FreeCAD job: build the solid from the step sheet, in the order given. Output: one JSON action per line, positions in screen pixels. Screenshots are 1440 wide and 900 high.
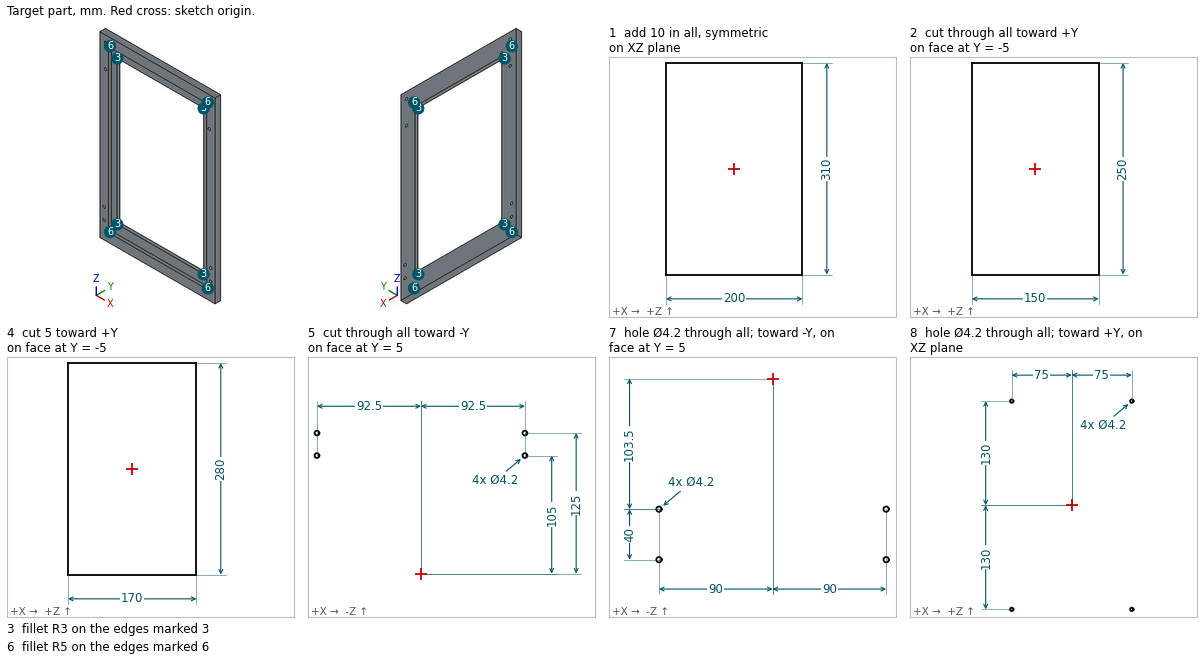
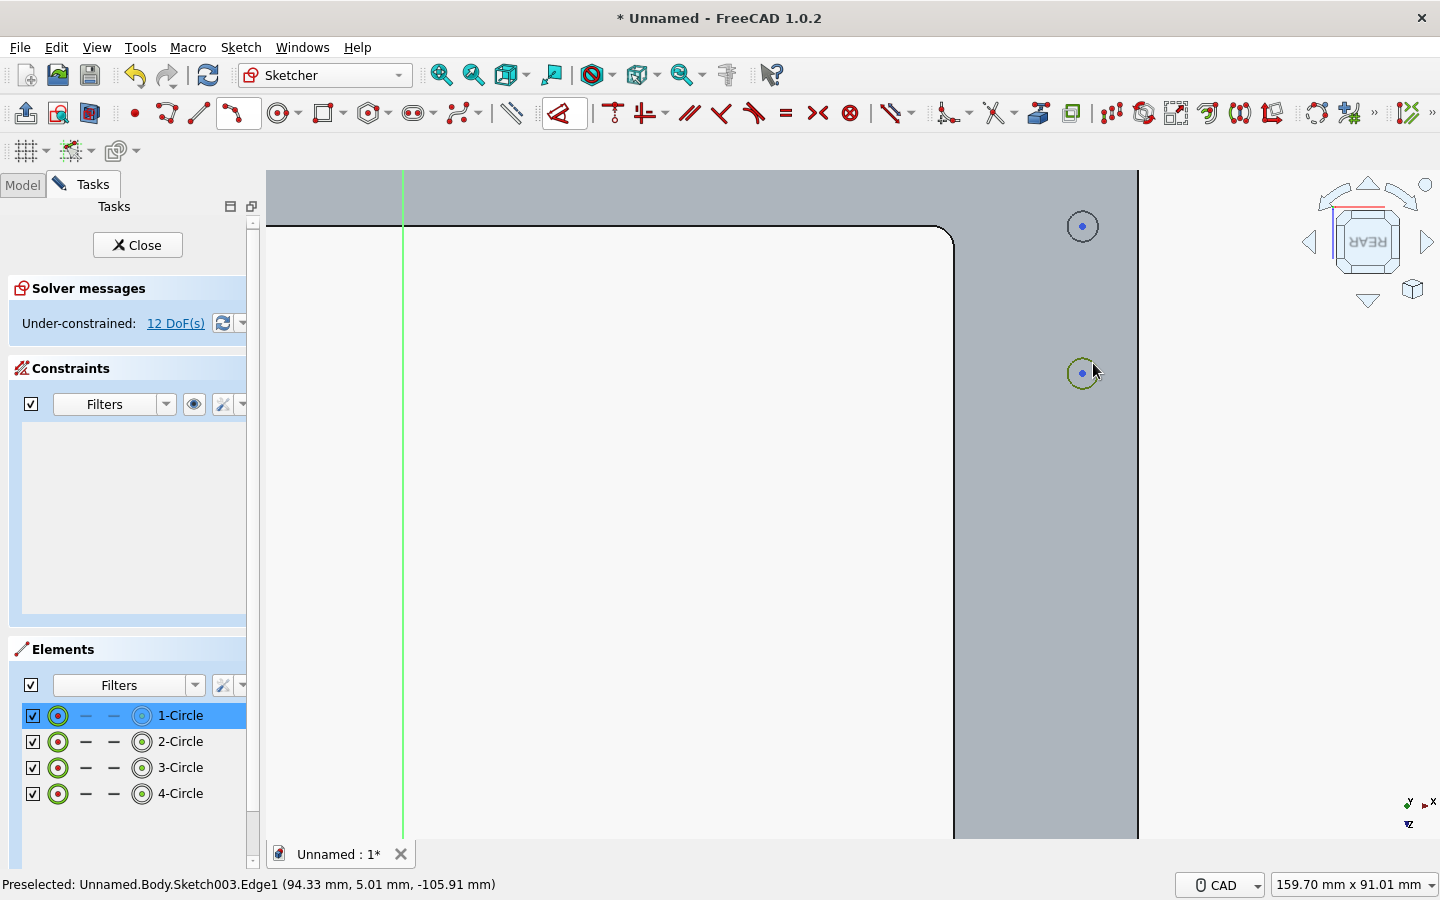
{"action": "left_click", "coordinate": [1093, 216]}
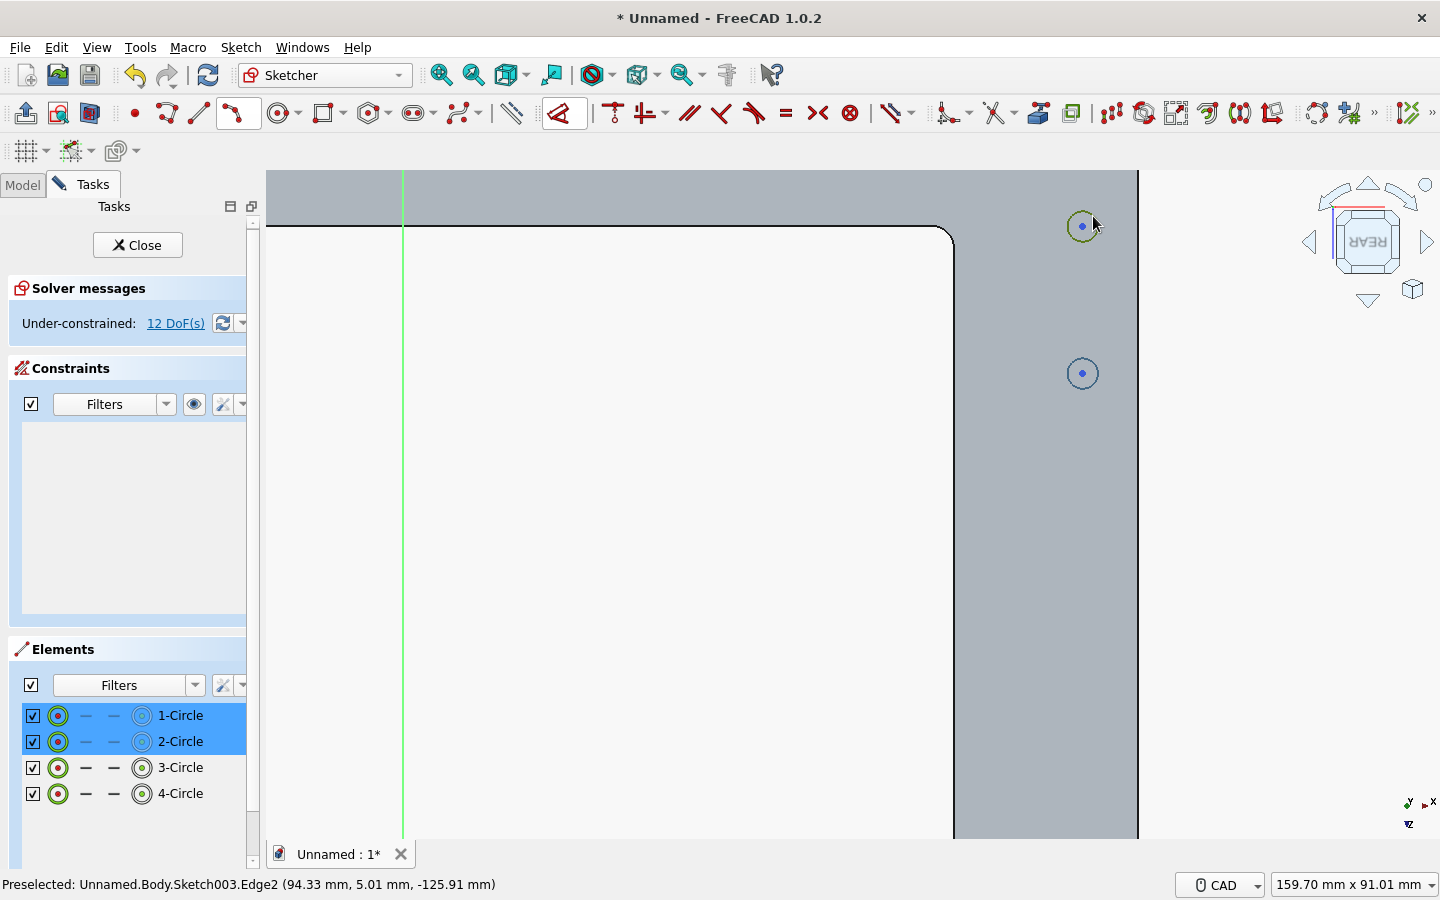
{"action": "scroll", "coordinate": [1096, 363], "scroll_direction": "down", "scroll_amount": 4}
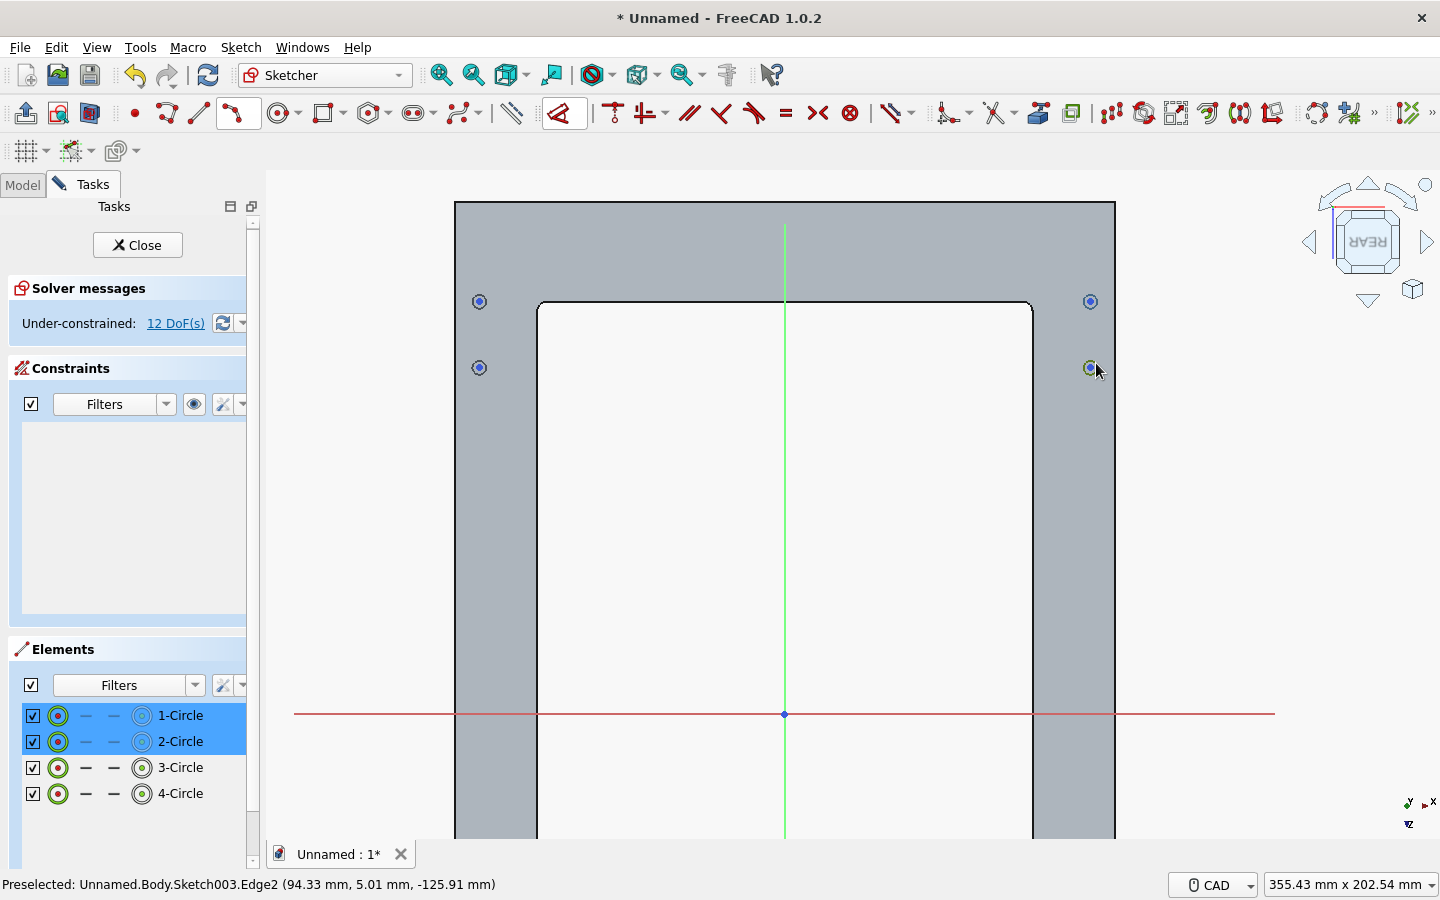
{"action": "scroll", "coordinate": [484, 363], "scroll_direction": "up", "scroll_amount": 4}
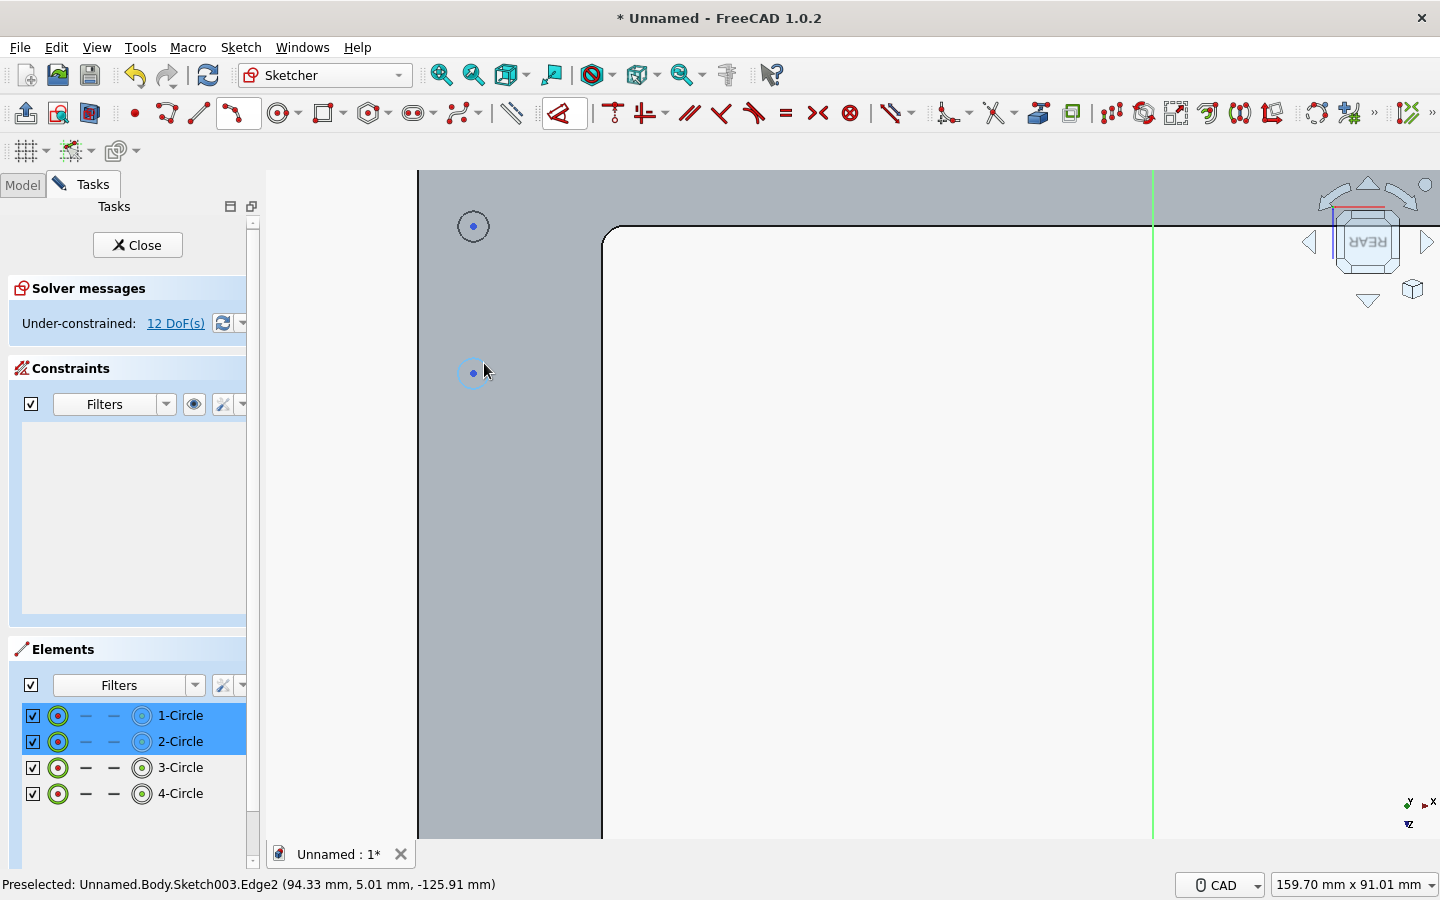
{"action": "left_click", "coordinate": [484, 363]}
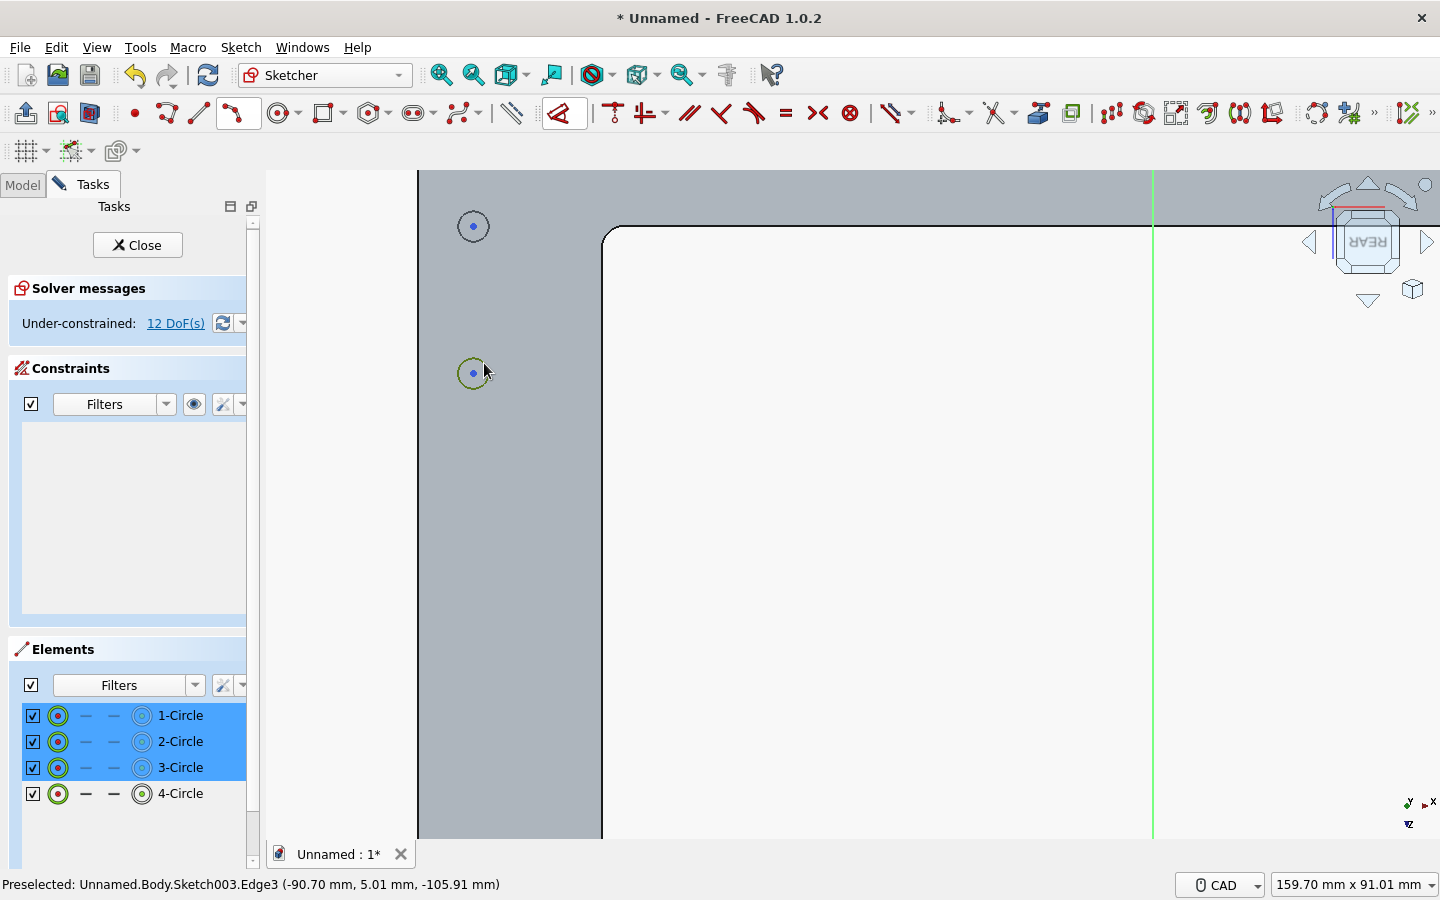
{"action": "left_click", "coordinate": [484, 216]}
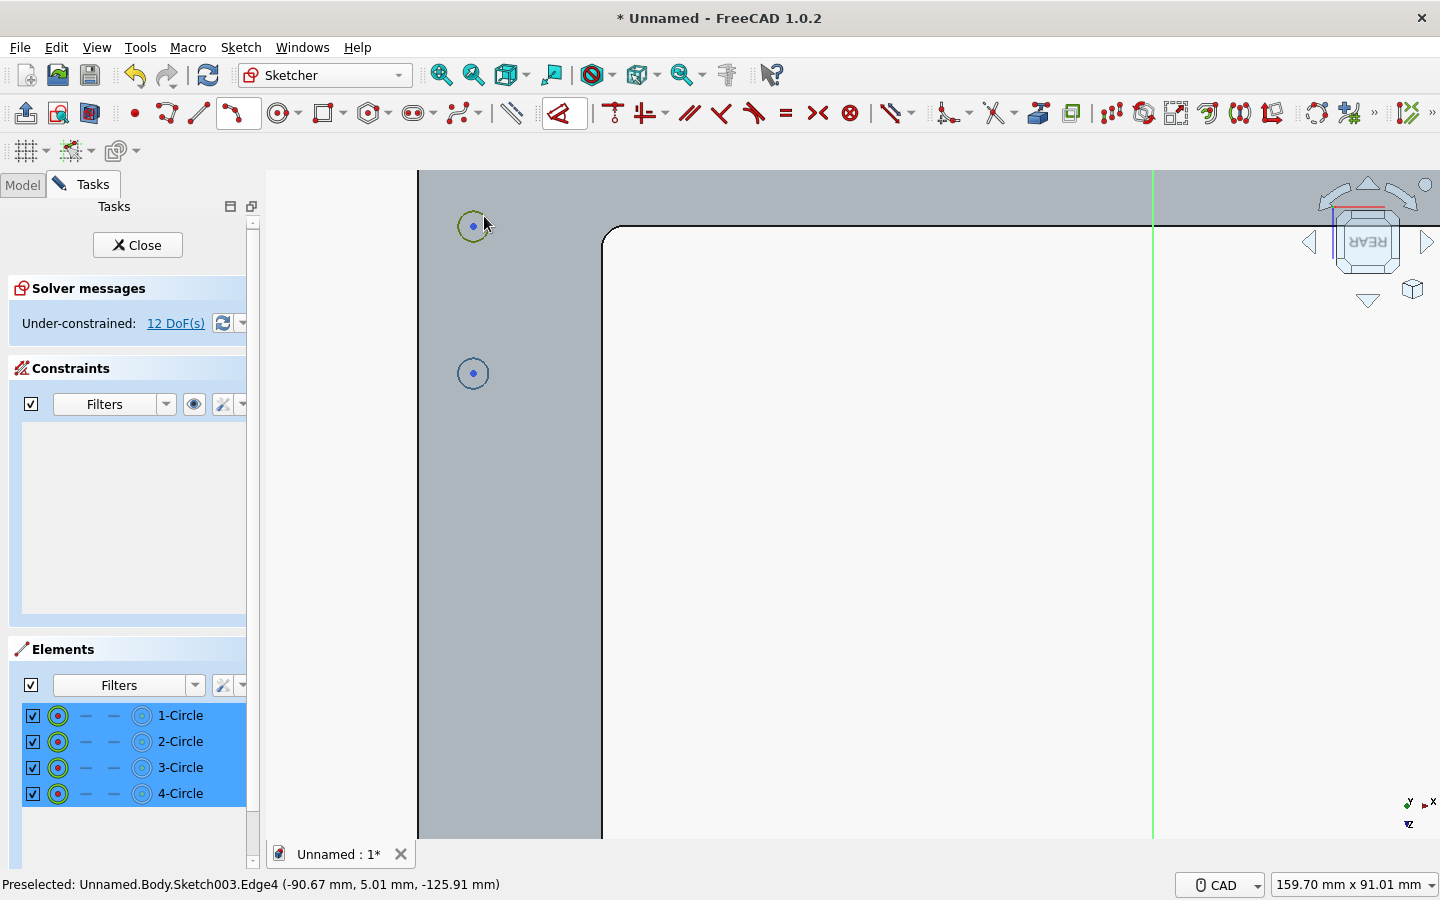
{"action": "left_click", "coordinate": [786, 114]}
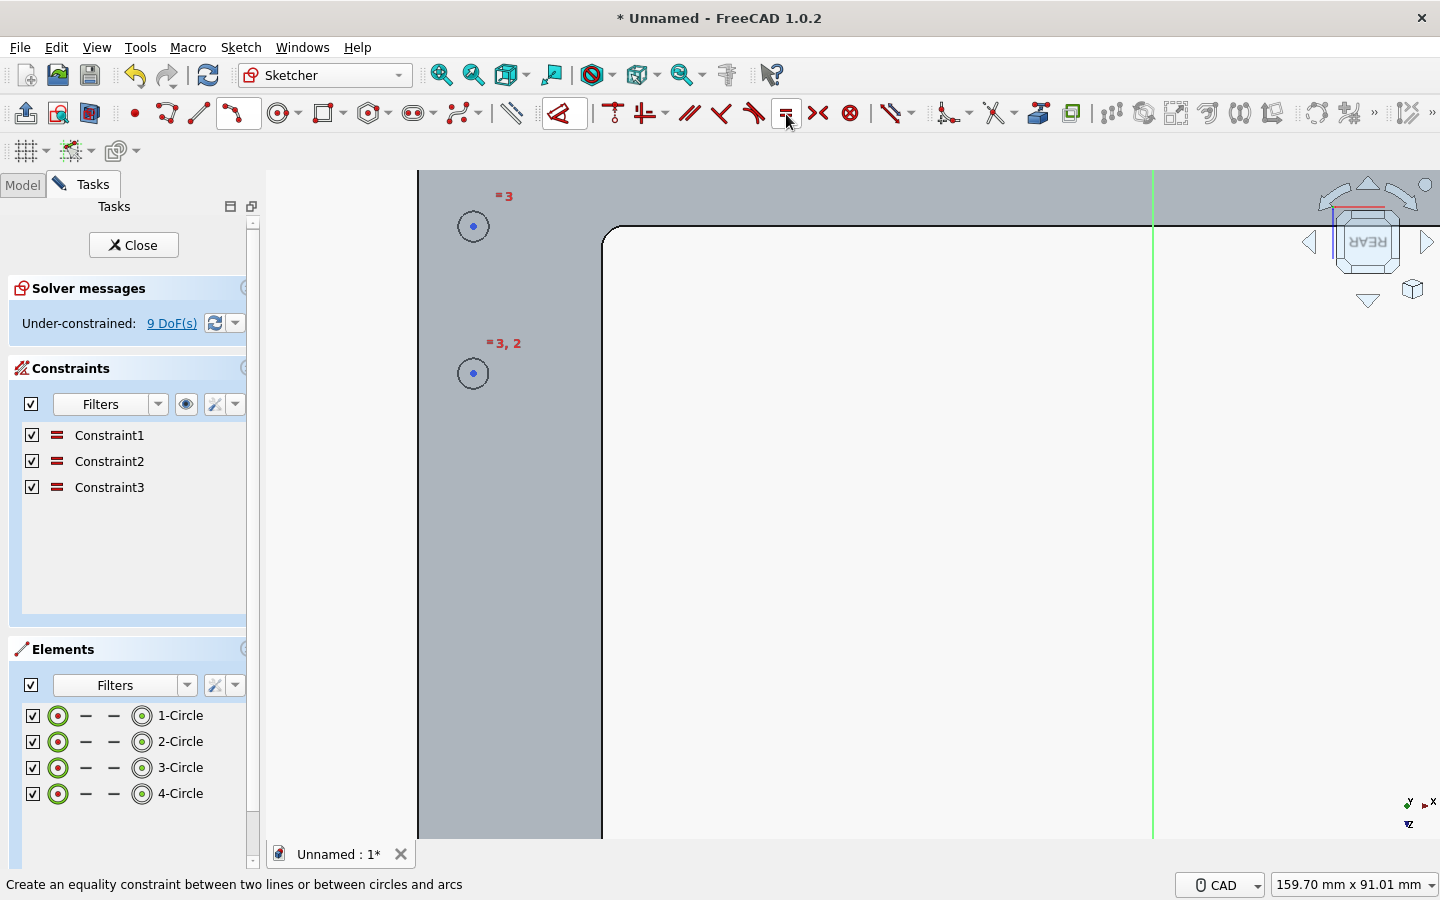
{"action": "scroll", "coordinate": [484, 363], "scroll_direction": "down", "scroll_amount": 4}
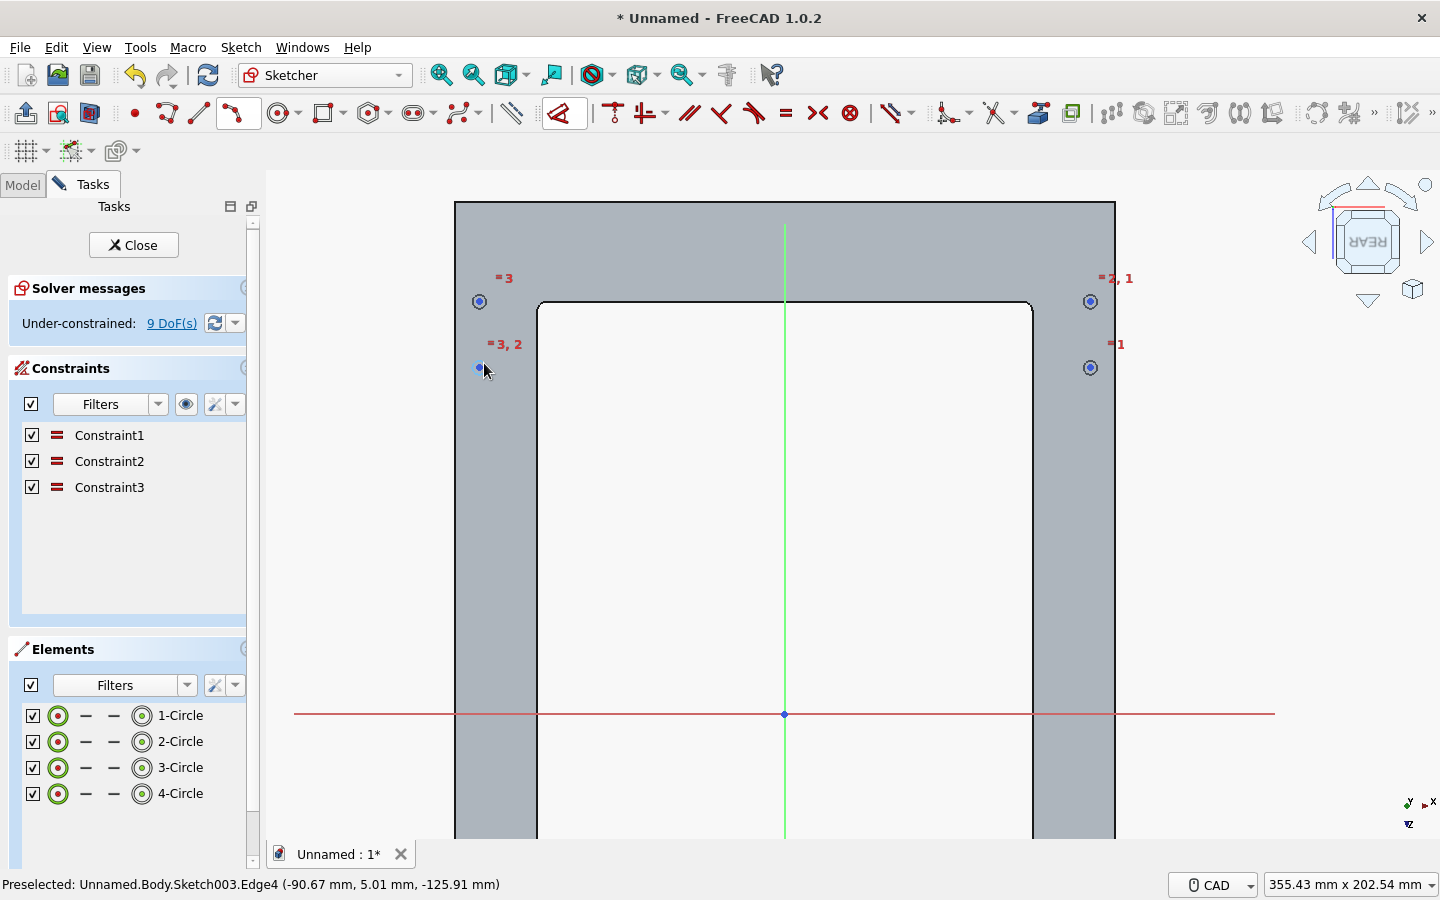
{"action": "left_click", "coordinate": [1090, 368]}